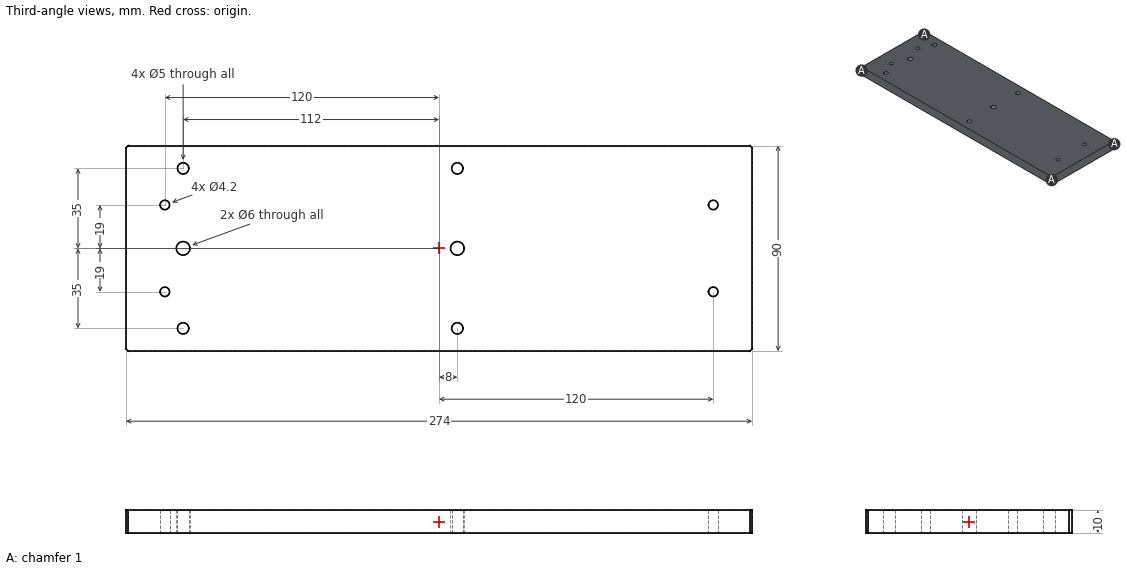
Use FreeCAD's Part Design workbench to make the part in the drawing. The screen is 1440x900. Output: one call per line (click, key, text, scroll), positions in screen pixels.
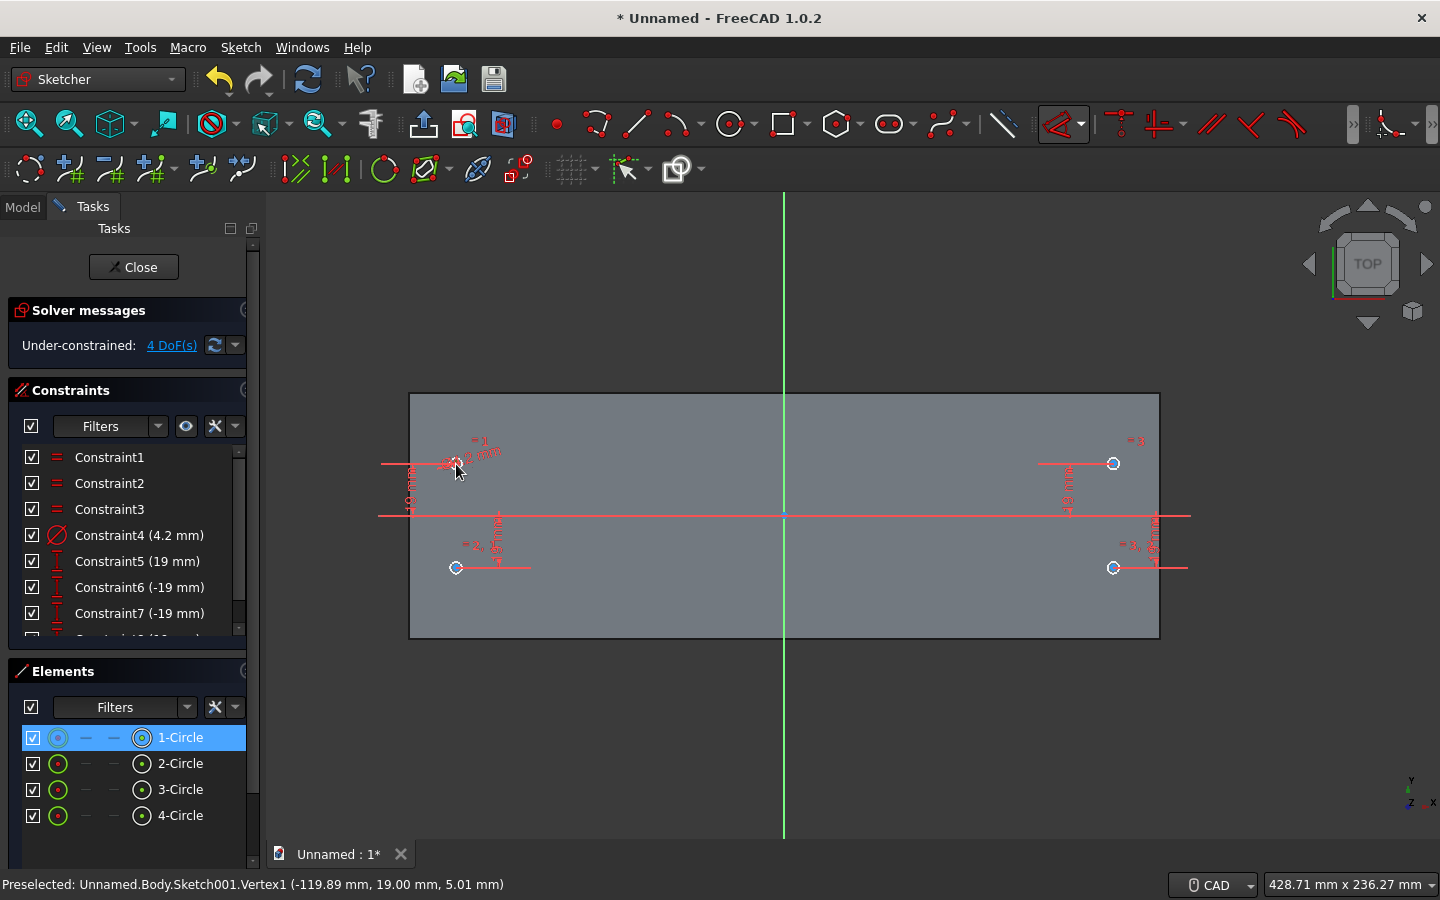
key(l)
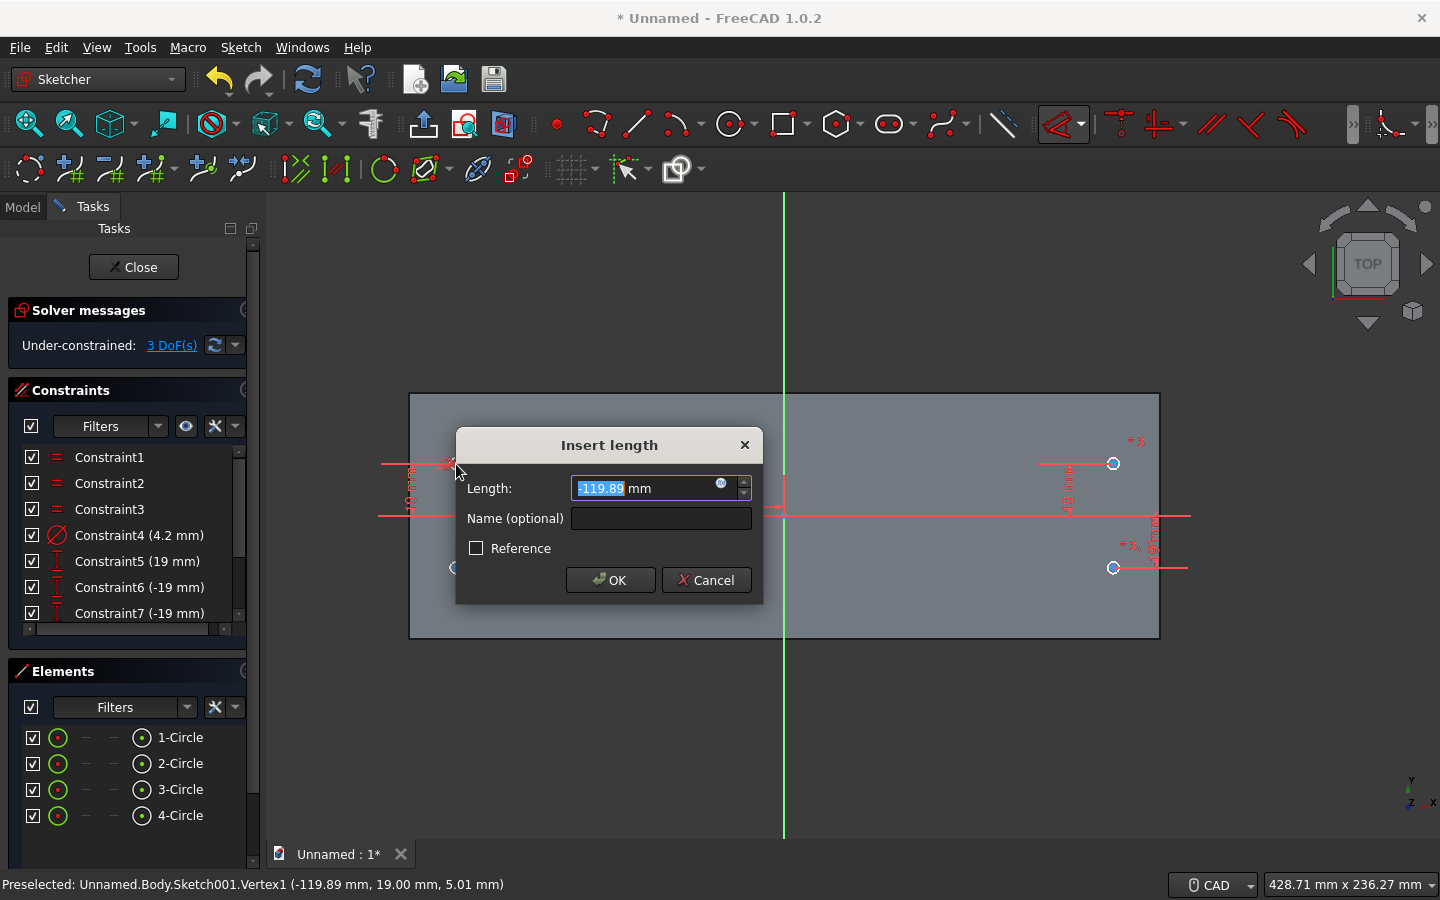
text(-120)
key(Return)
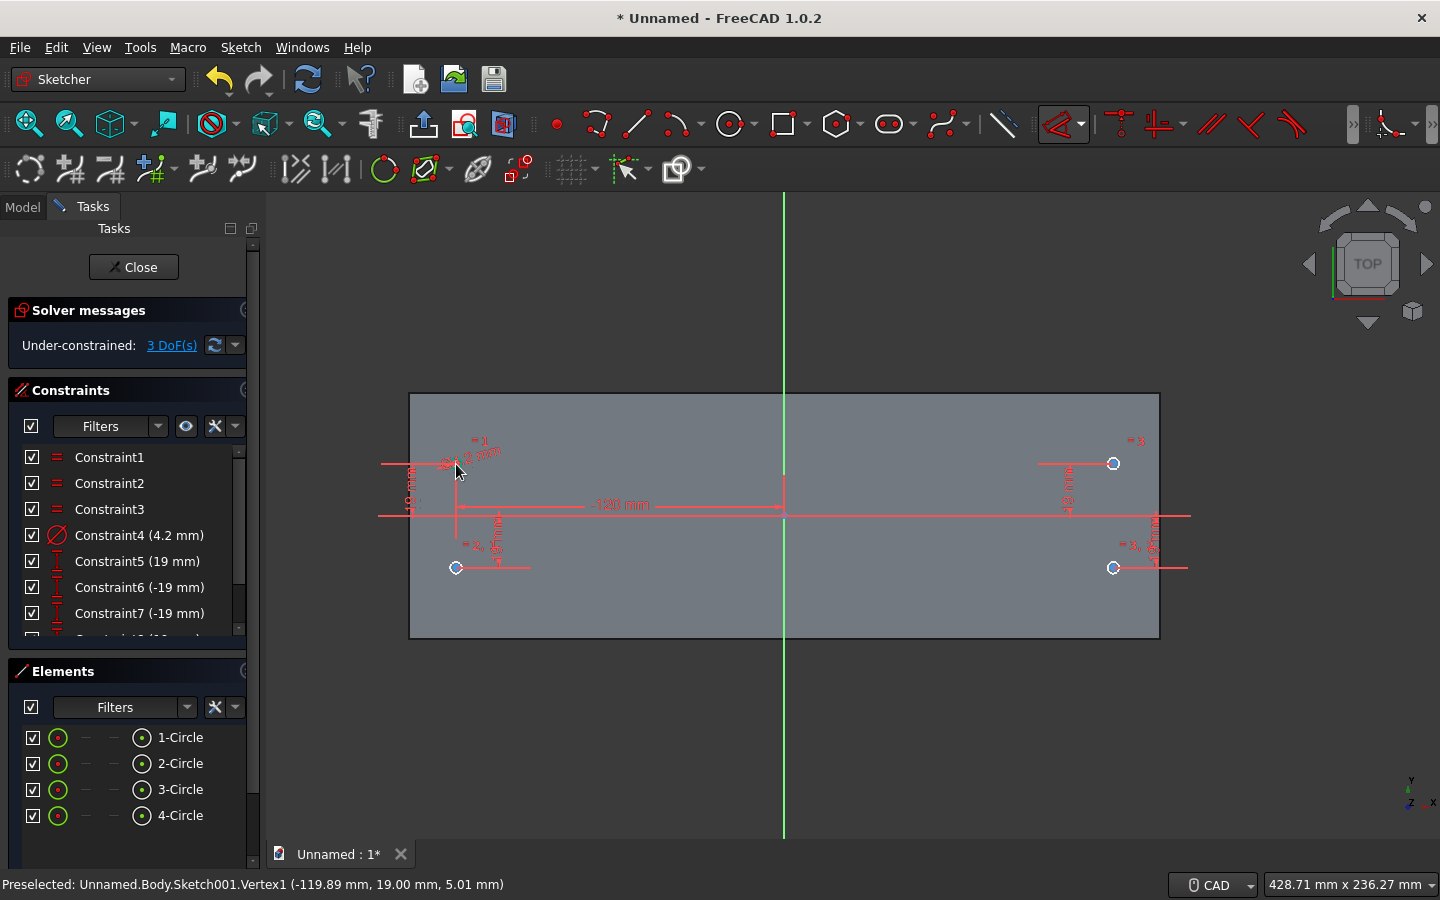
click(456, 568)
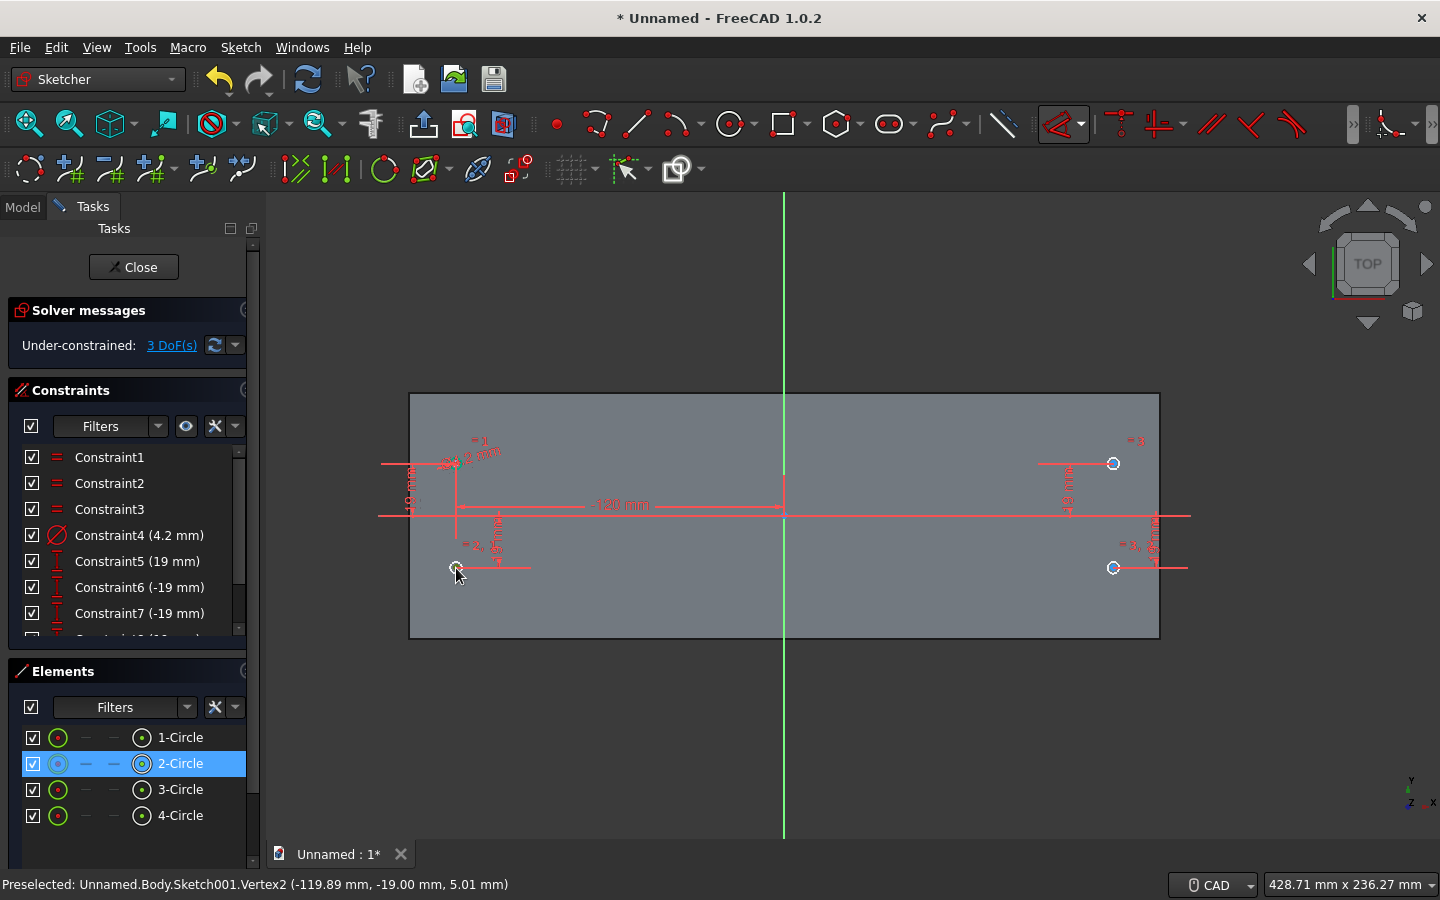
click(1084, 124)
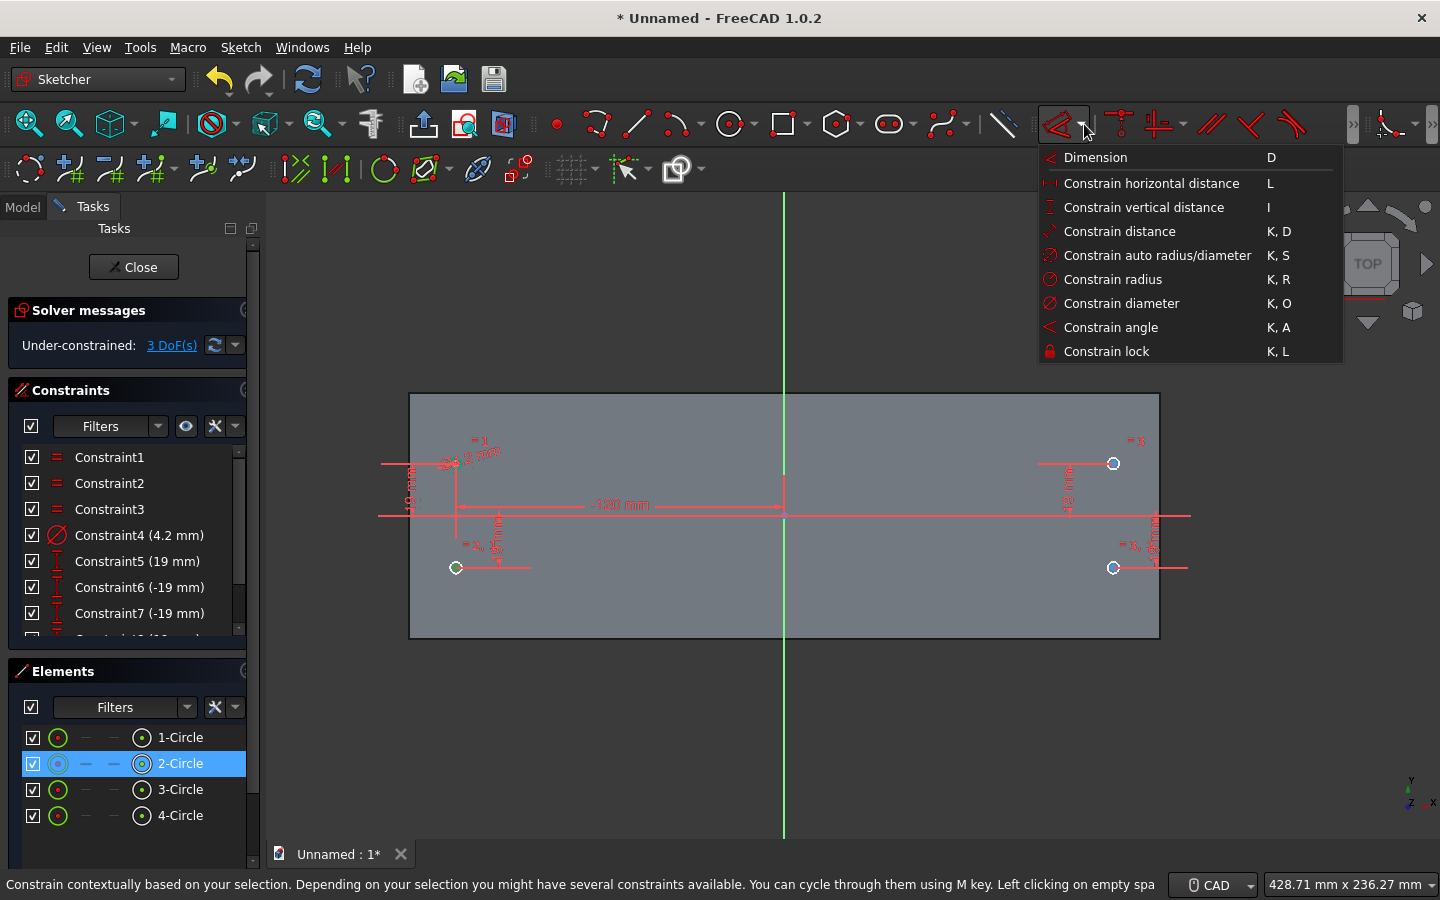
click(1191, 183)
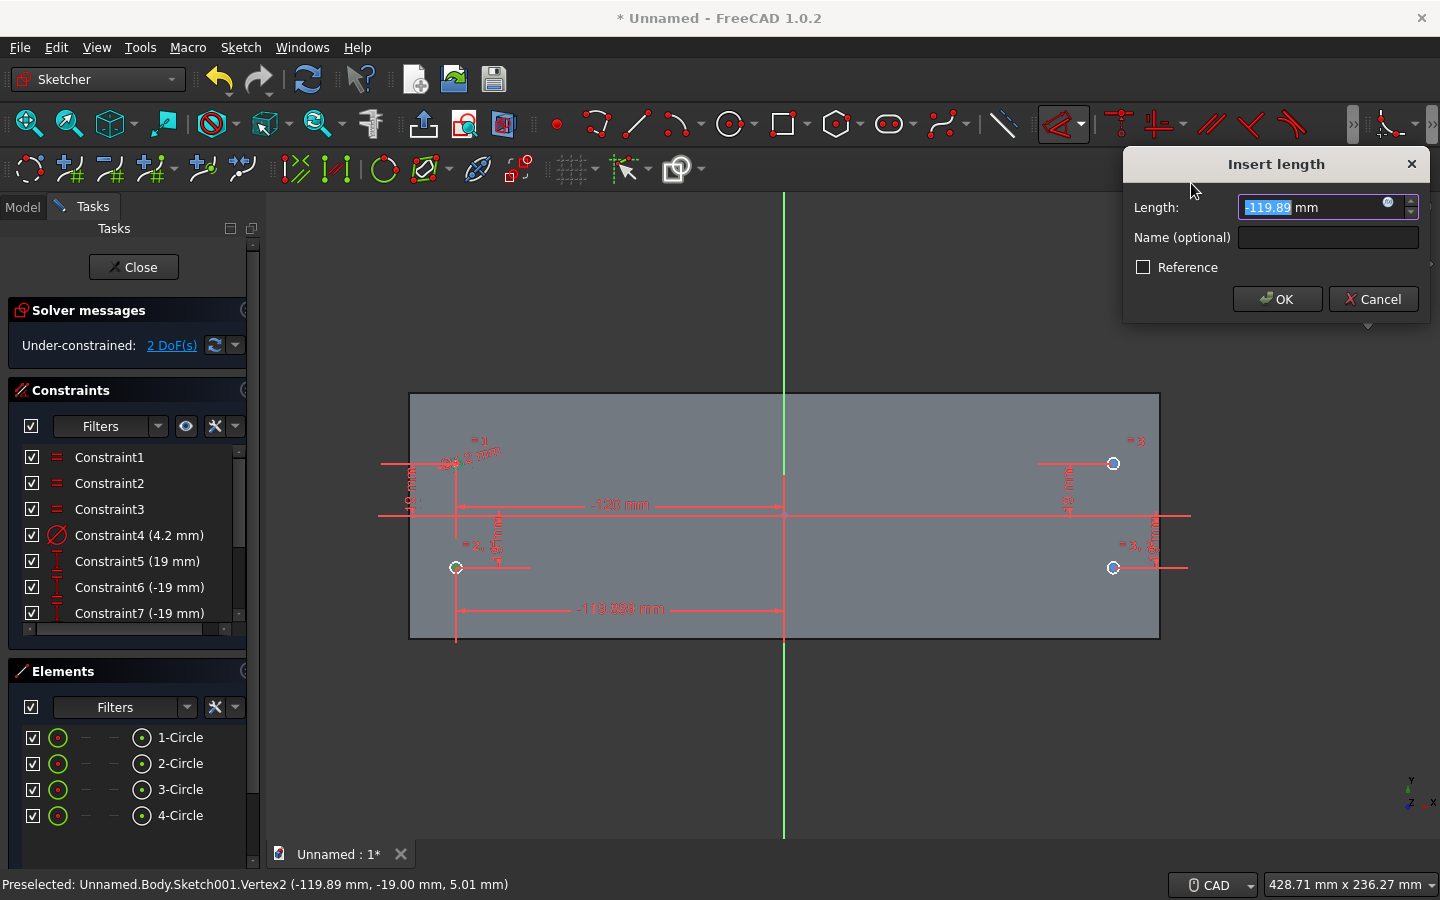
text(-120)
key(Return)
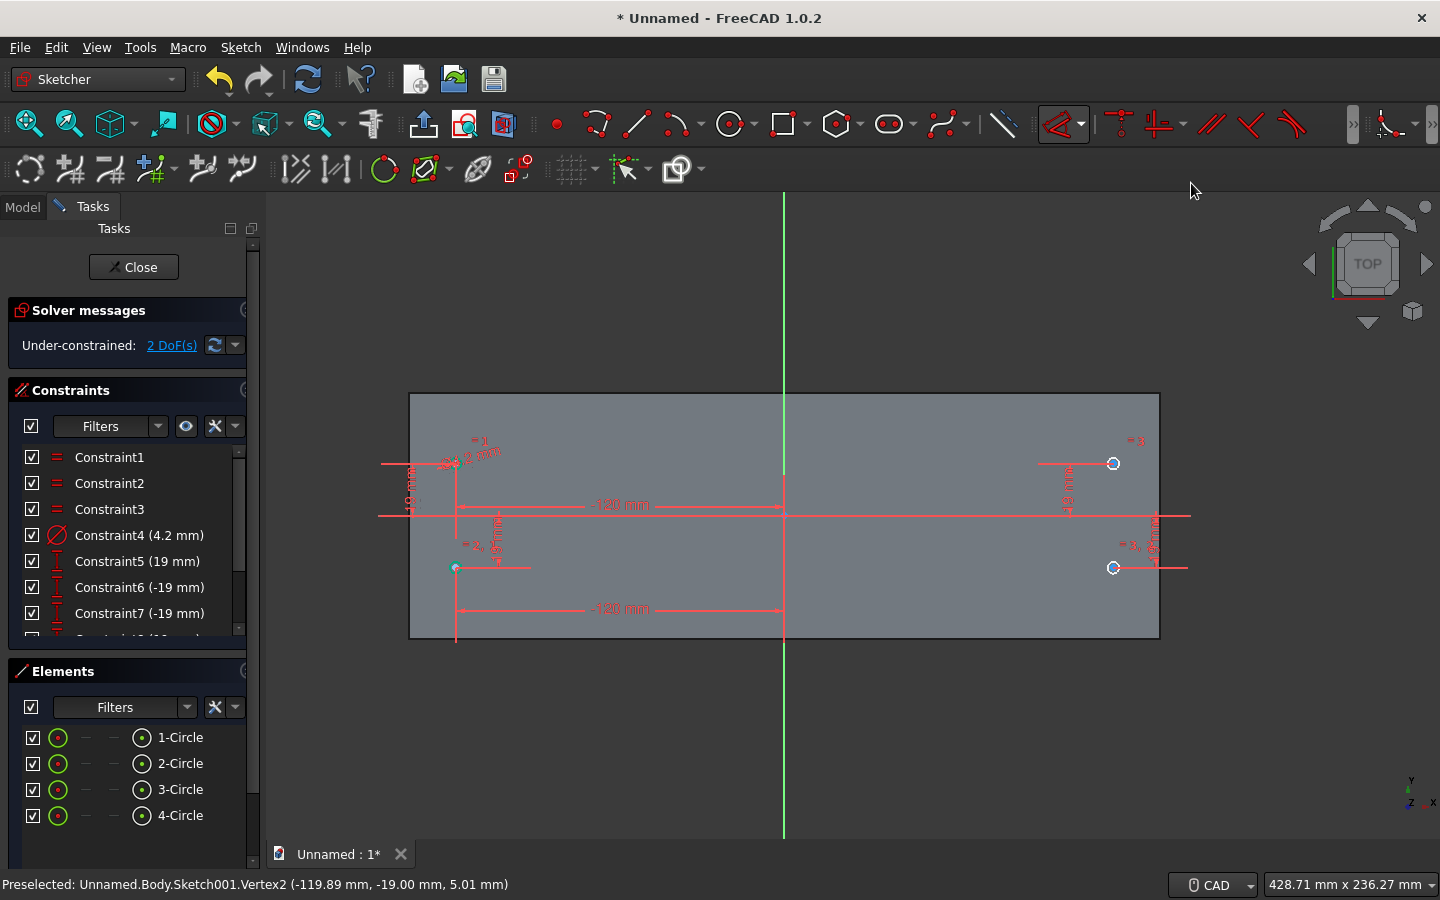
click(1113, 568)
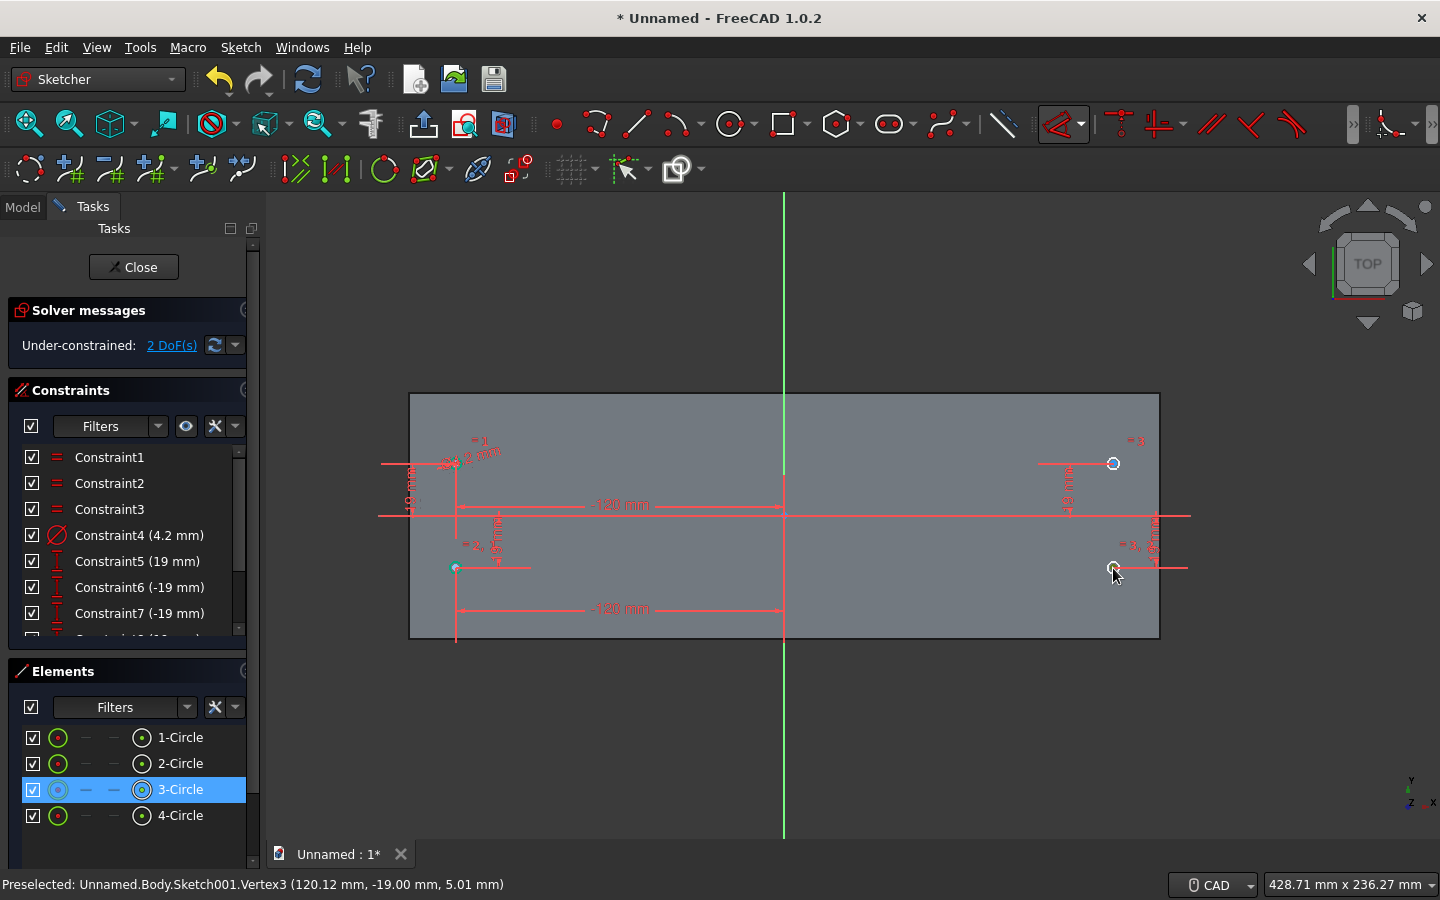
key(l)